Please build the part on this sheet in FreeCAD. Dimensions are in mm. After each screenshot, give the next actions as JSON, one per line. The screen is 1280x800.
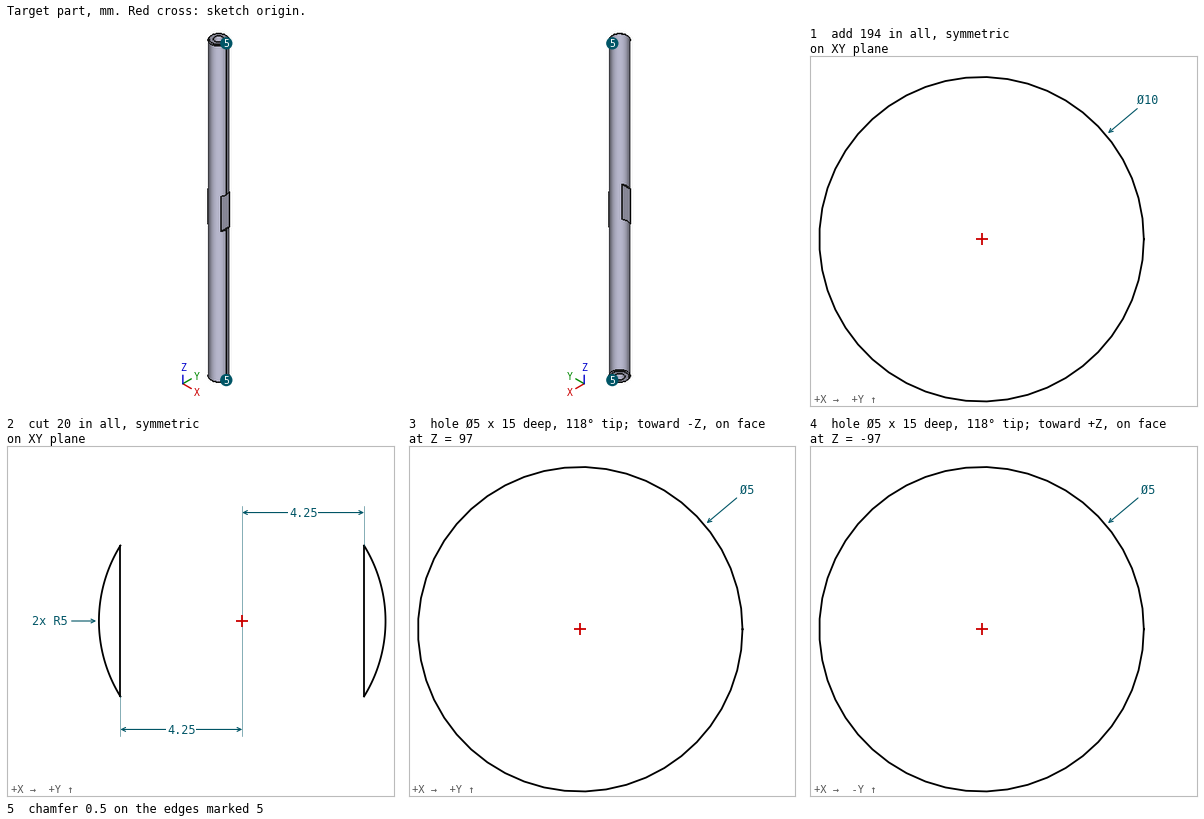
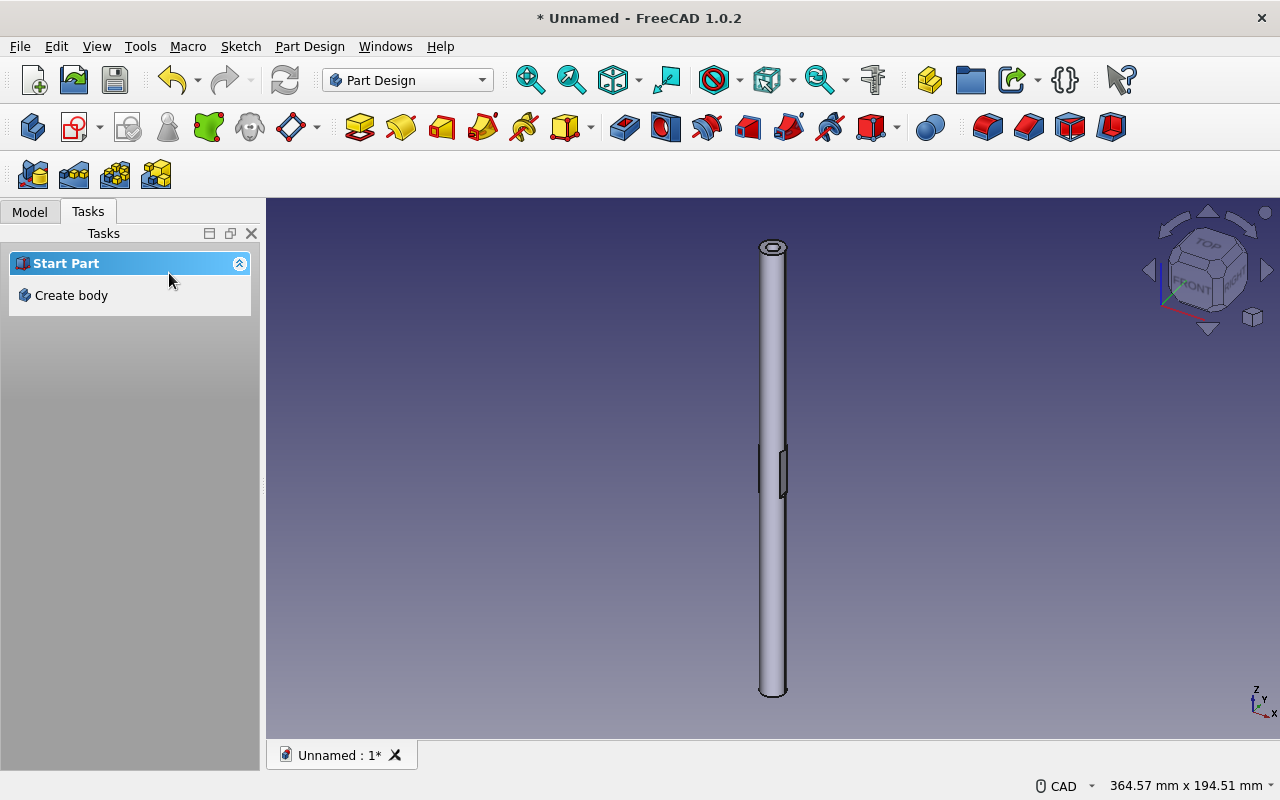
{"action": "key", "text": "5"}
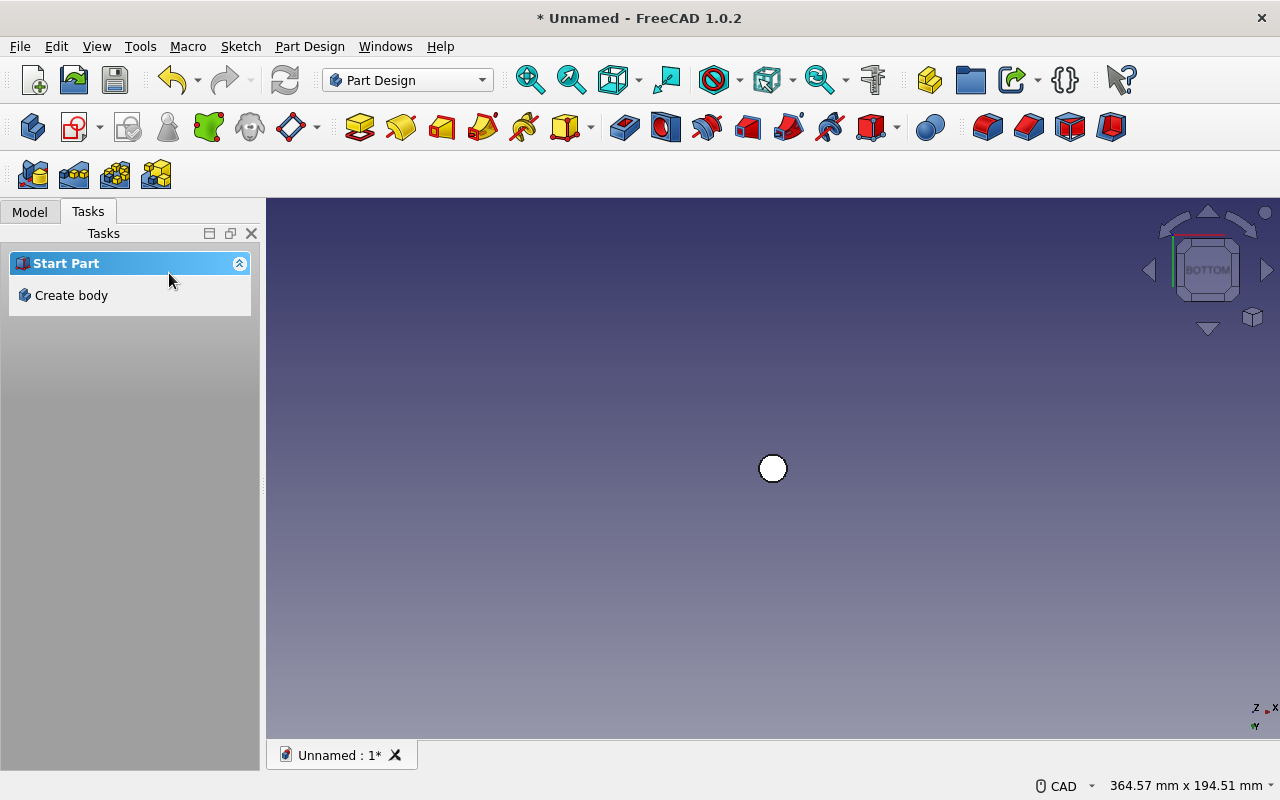
{"action": "left_click", "coordinate": [531, 80]}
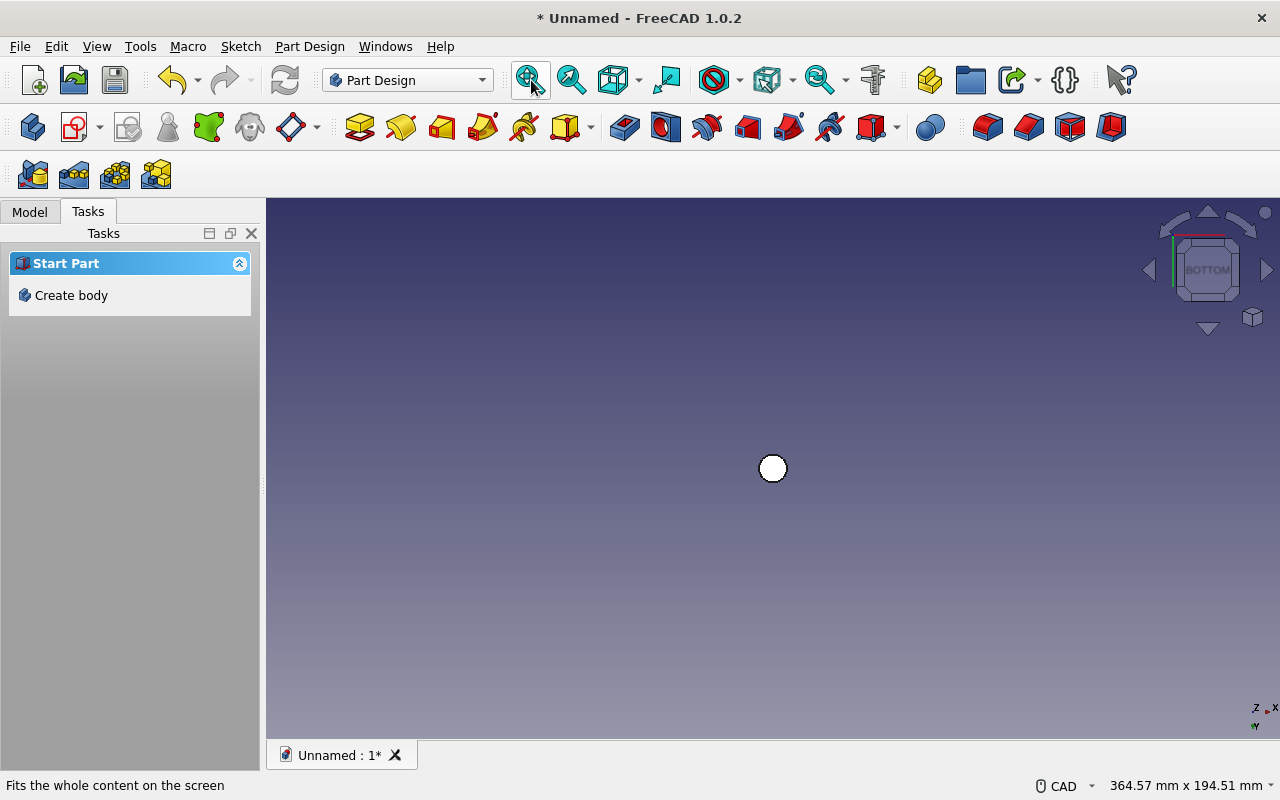
{"action": "left_click", "coordinate": [773, 467]}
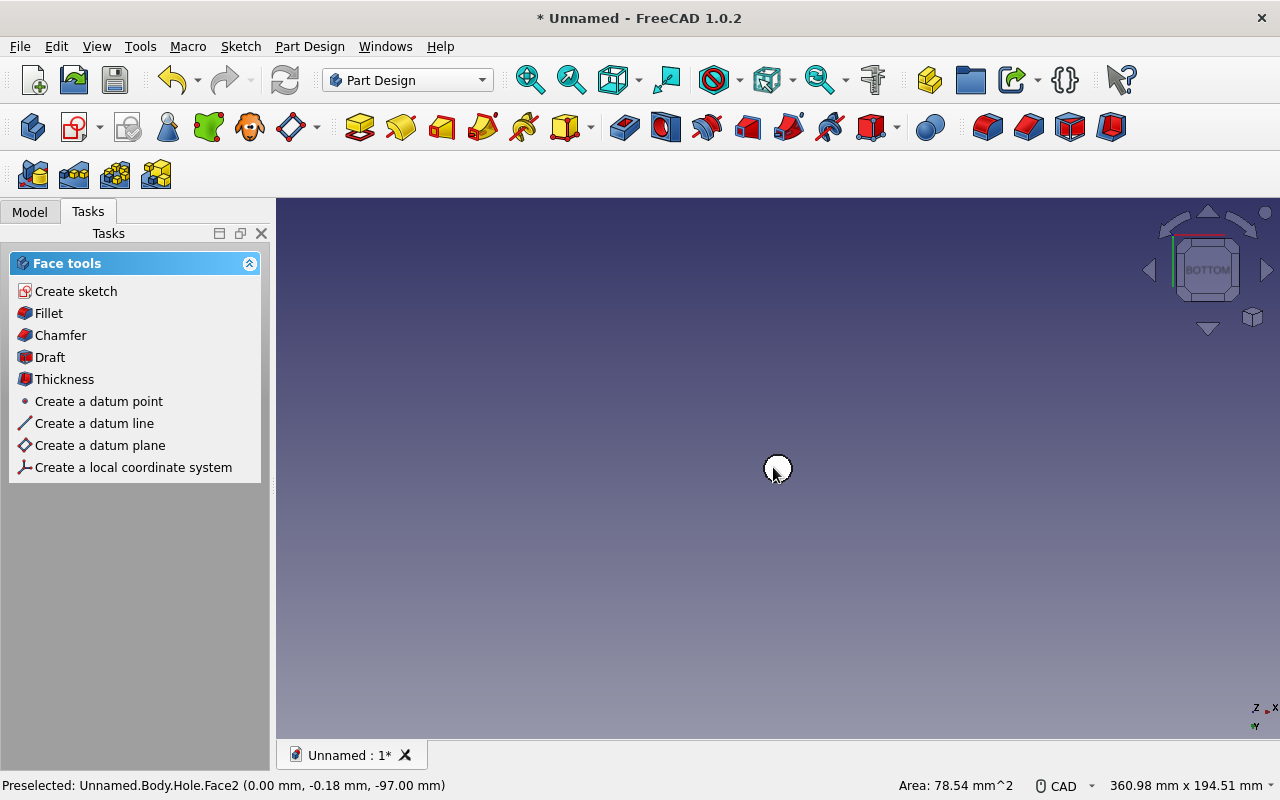
{"action": "left_click", "coordinate": [74, 128]}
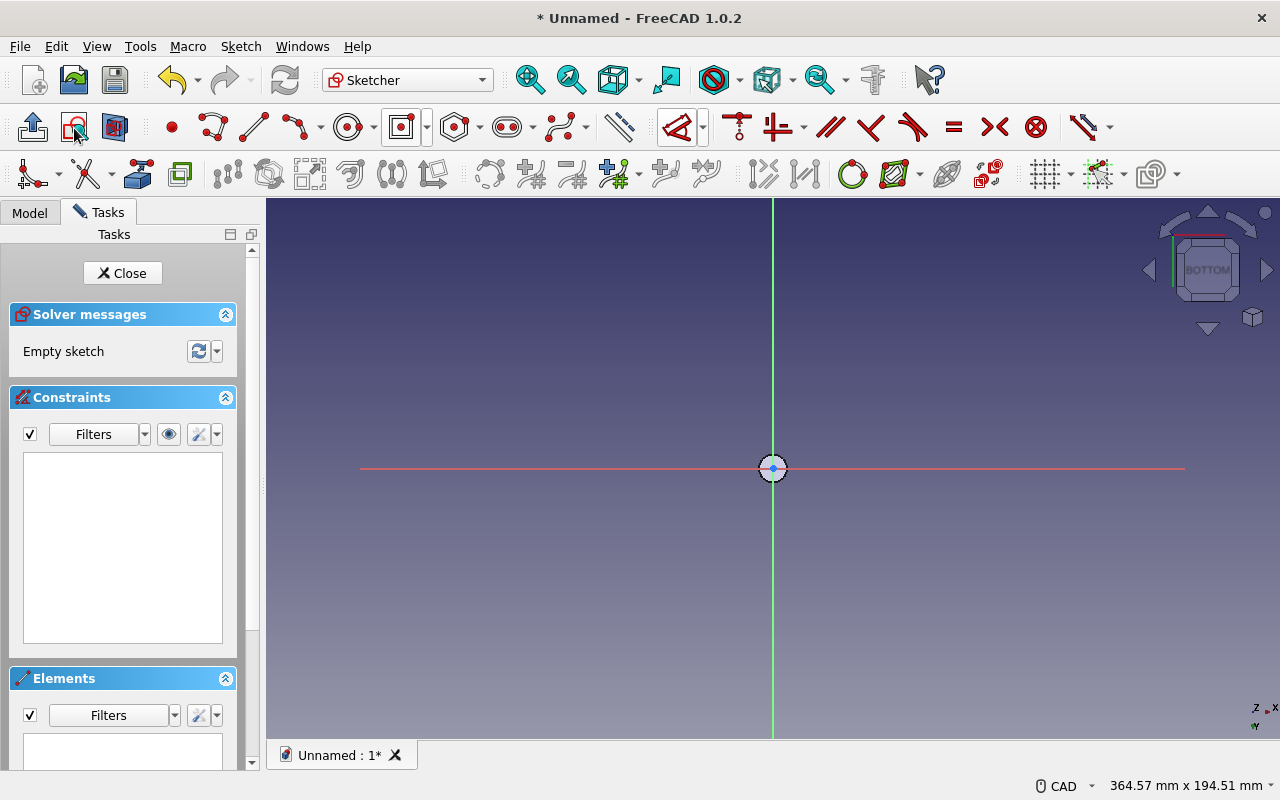
{"action": "scroll", "coordinate": [777, 468], "scroll_direction": "up", "scroll_amount": 15}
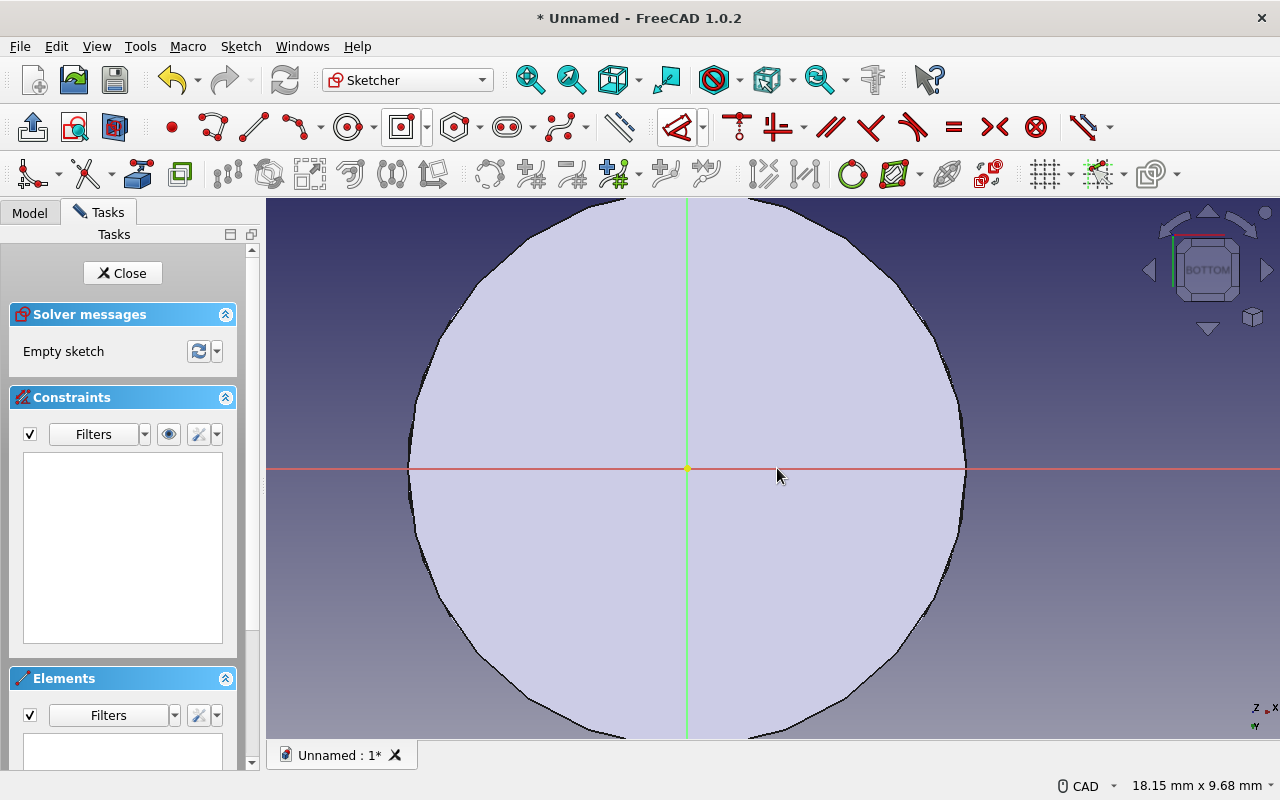
{"action": "left_click", "coordinate": [348, 128]}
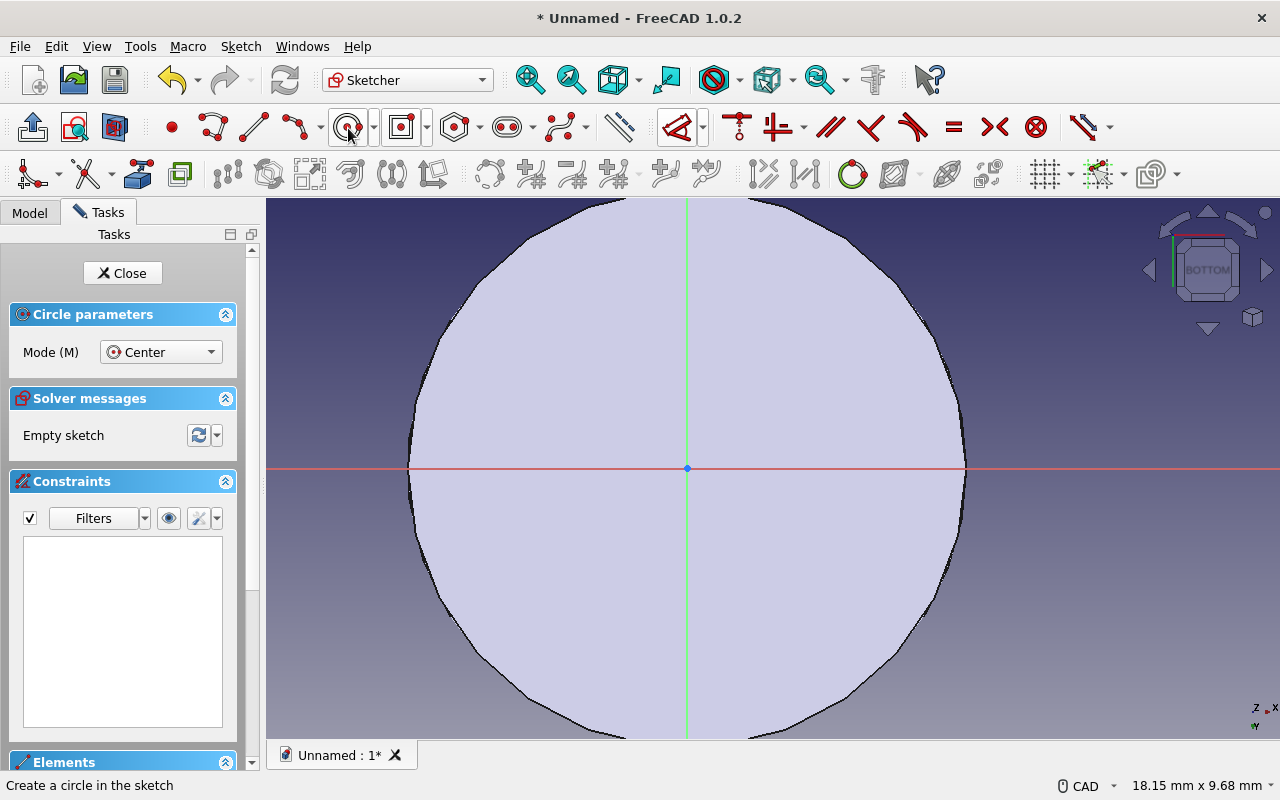
{"action": "left_click", "coordinate": [687, 468]}
{"action": "left_click", "coordinate": [786, 370]}
{"action": "key", "text": "Escape"}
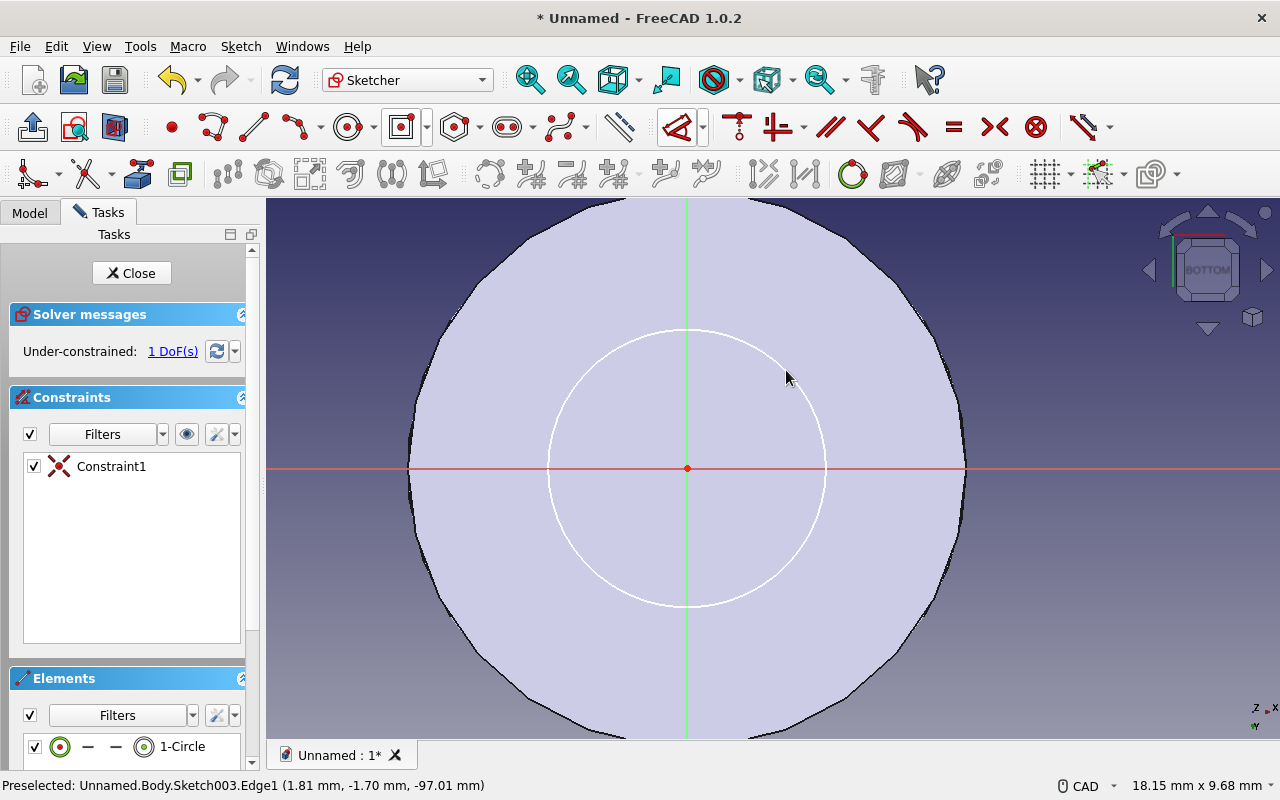
{"action": "left_click", "coordinate": [785, 370]}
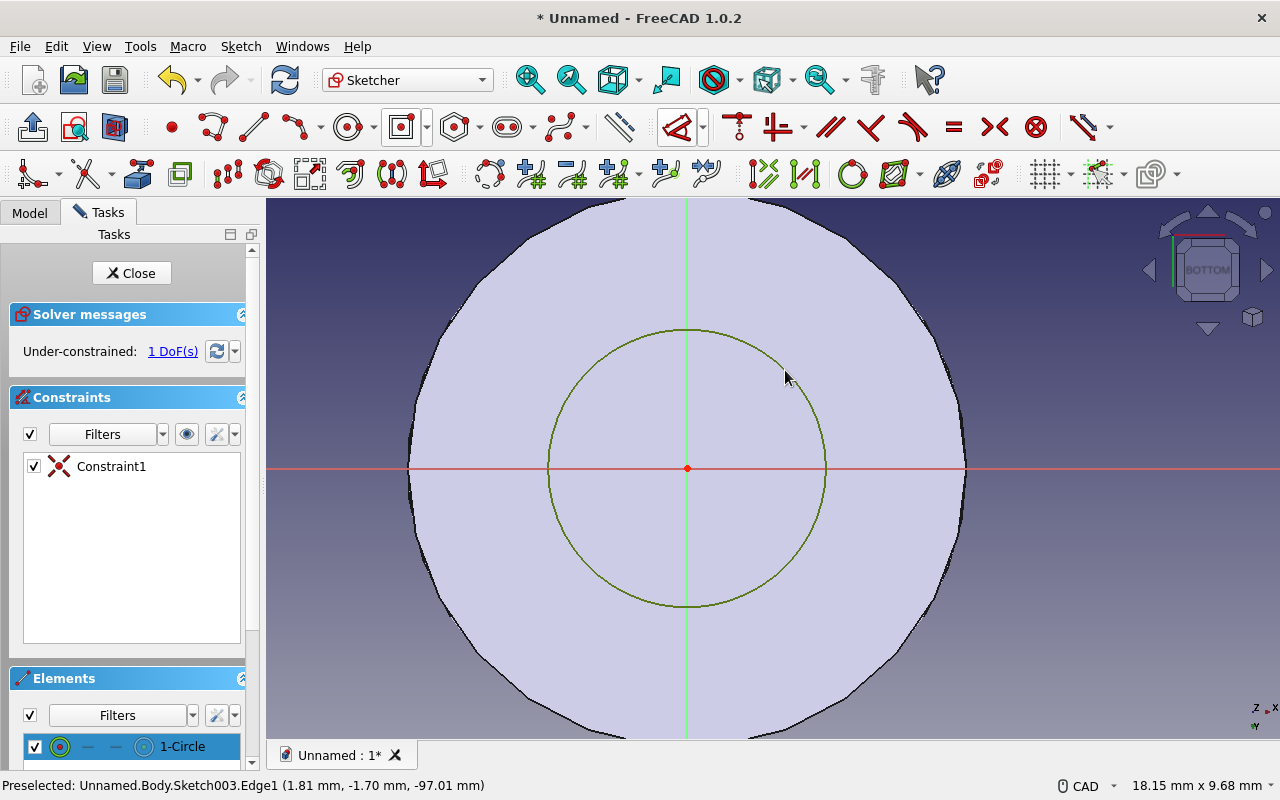
{"action": "left_click", "coordinate": [702, 128]}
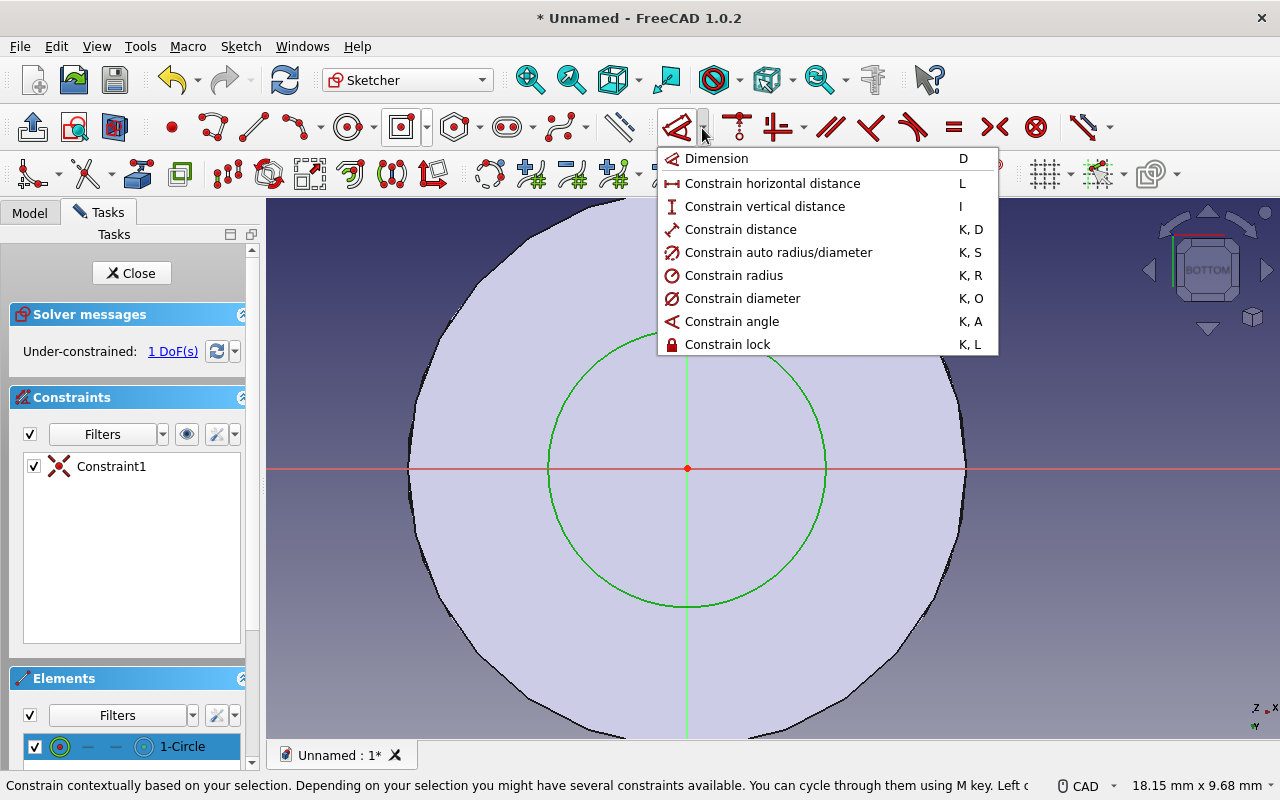
{"action": "left_click", "coordinate": [828, 298]}